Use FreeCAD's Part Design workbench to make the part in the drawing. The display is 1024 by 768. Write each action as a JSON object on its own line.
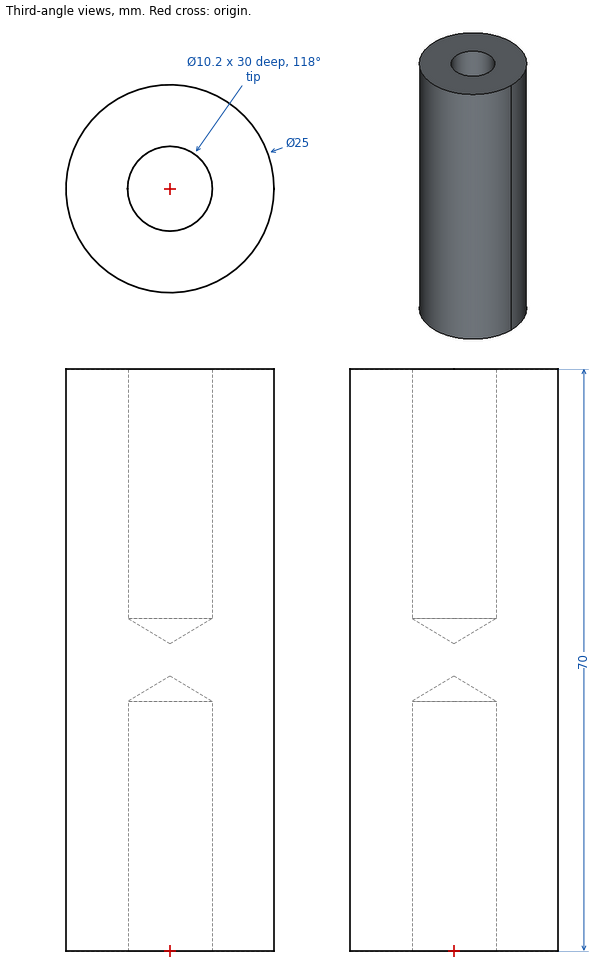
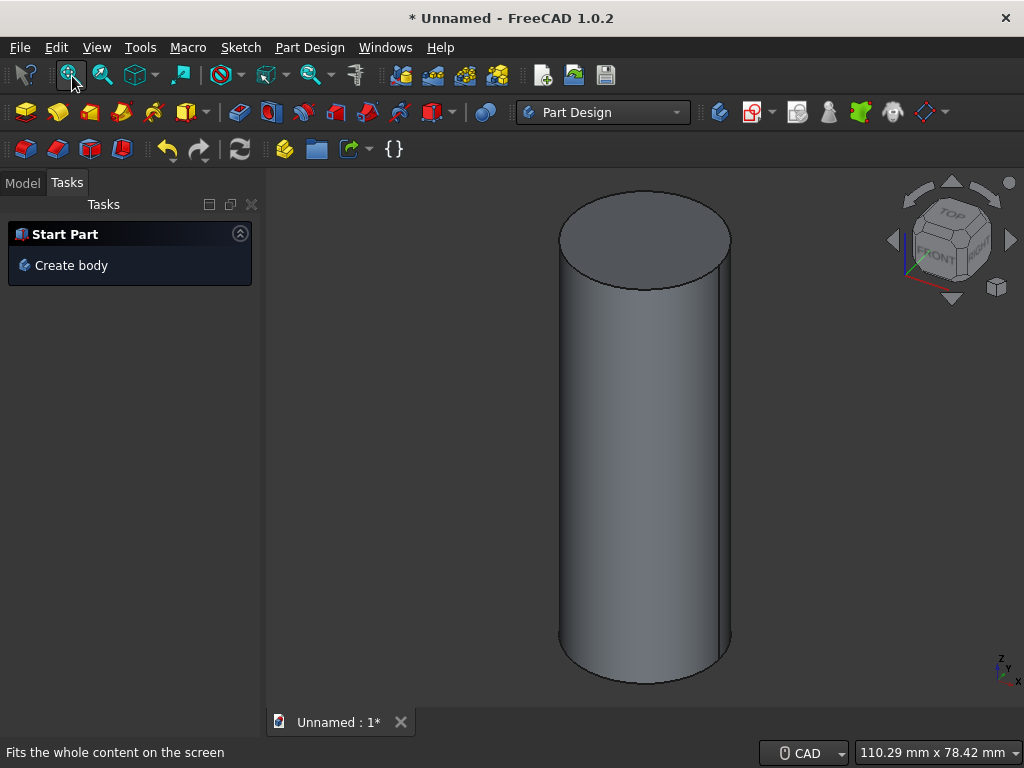
{"action": "left_click", "coordinate": [645, 239]}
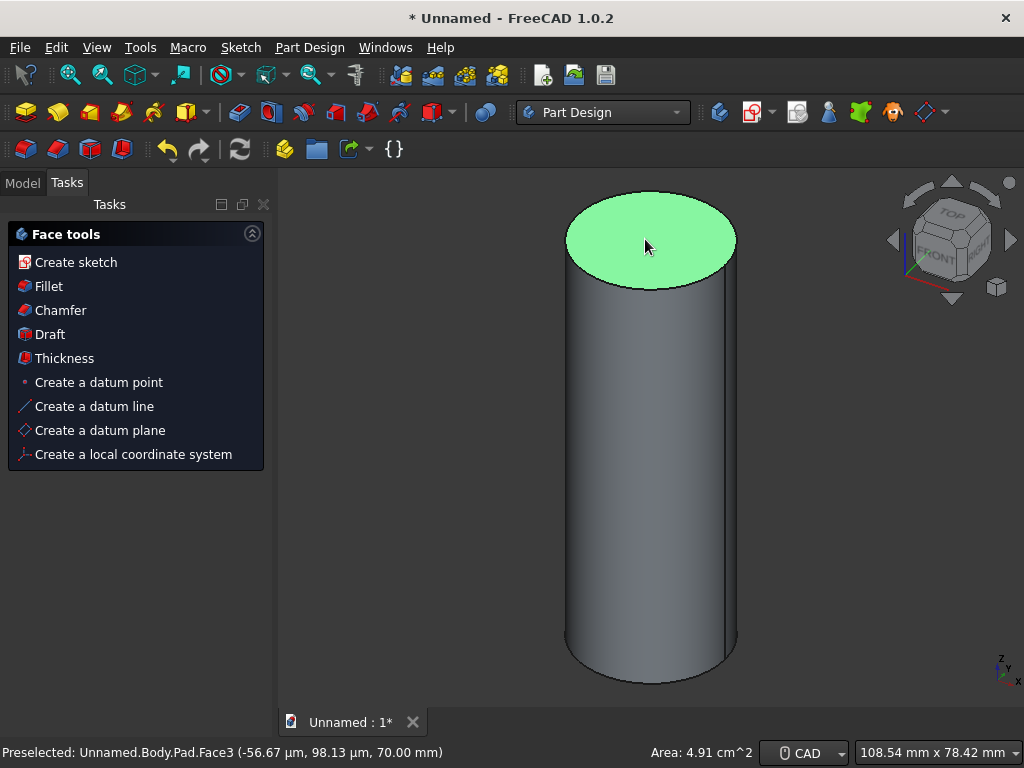
{"action": "left_click", "coordinate": [752, 112]}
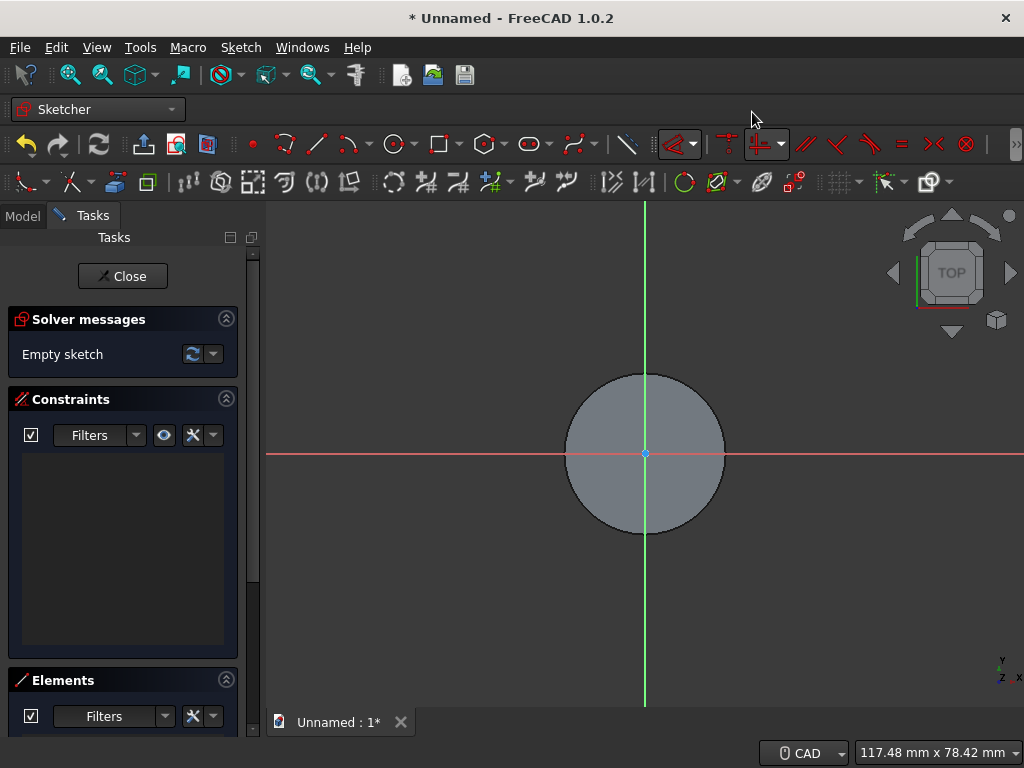
{"action": "scroll", "coordinate": [662, 454], "scroll_direction": "up", "scroll_amount": 8}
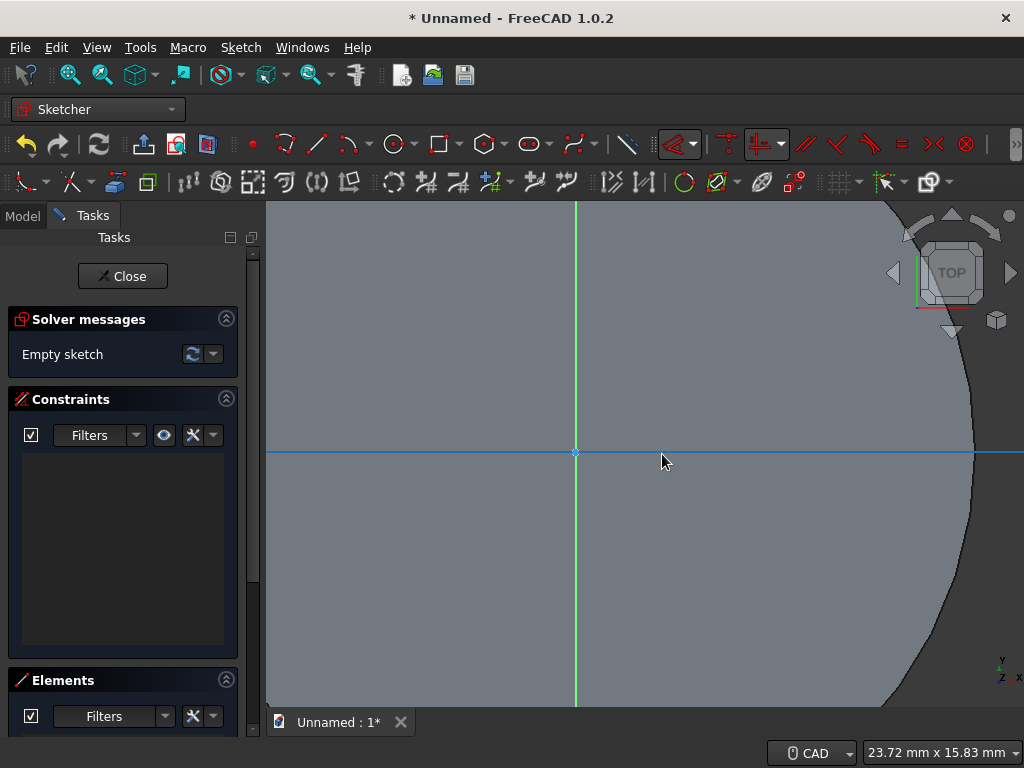
{"action": "key", "text": "g c"}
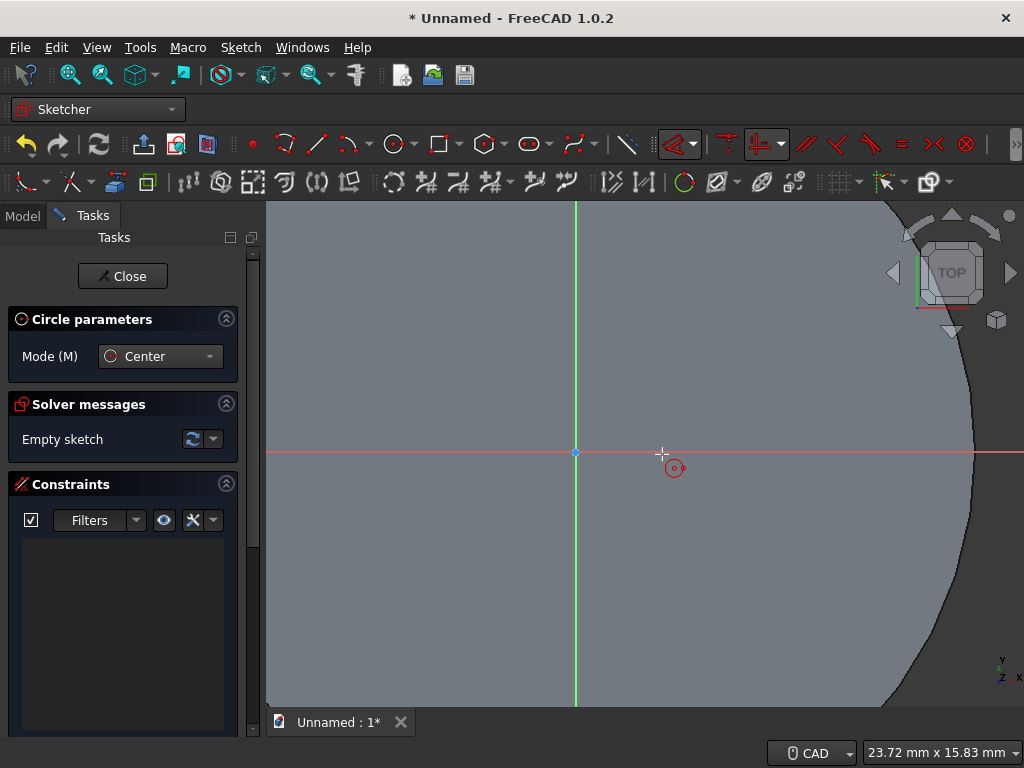
{"action": "left_click", "coordinate": [576, 452]}
{"action": "mouse_move", "coordinate": [691, 337]}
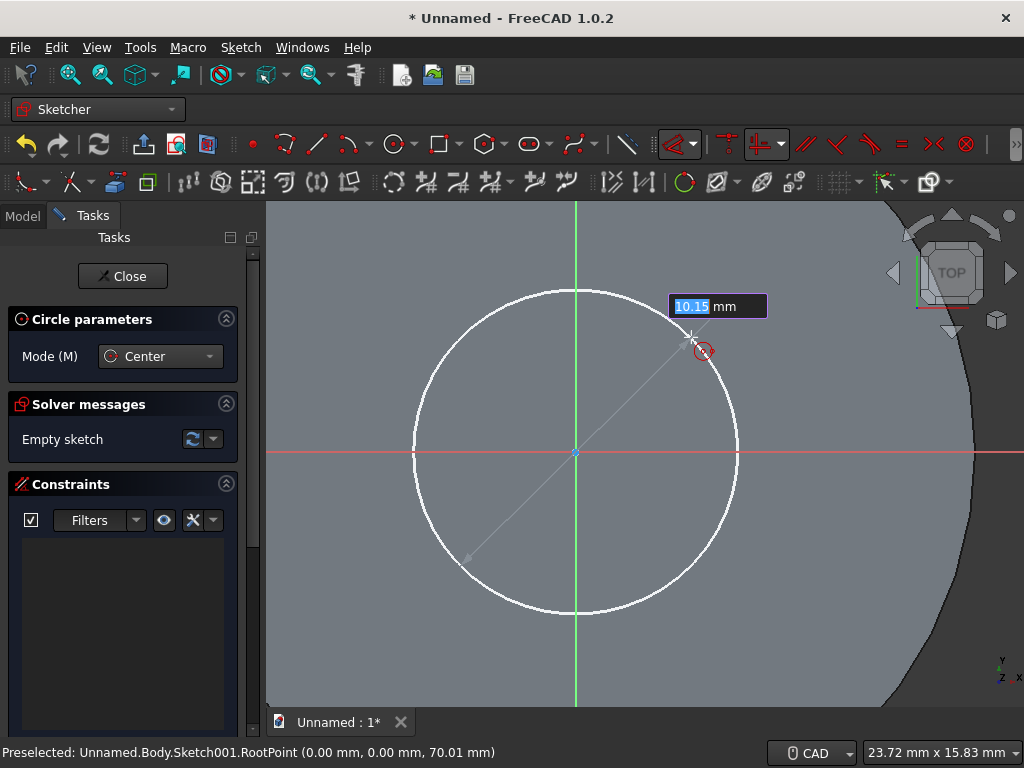
{"action": "type", "text": "10.2"}
{"action": "key", "text": "Return"}
{"action": "key", "text": "Escape"}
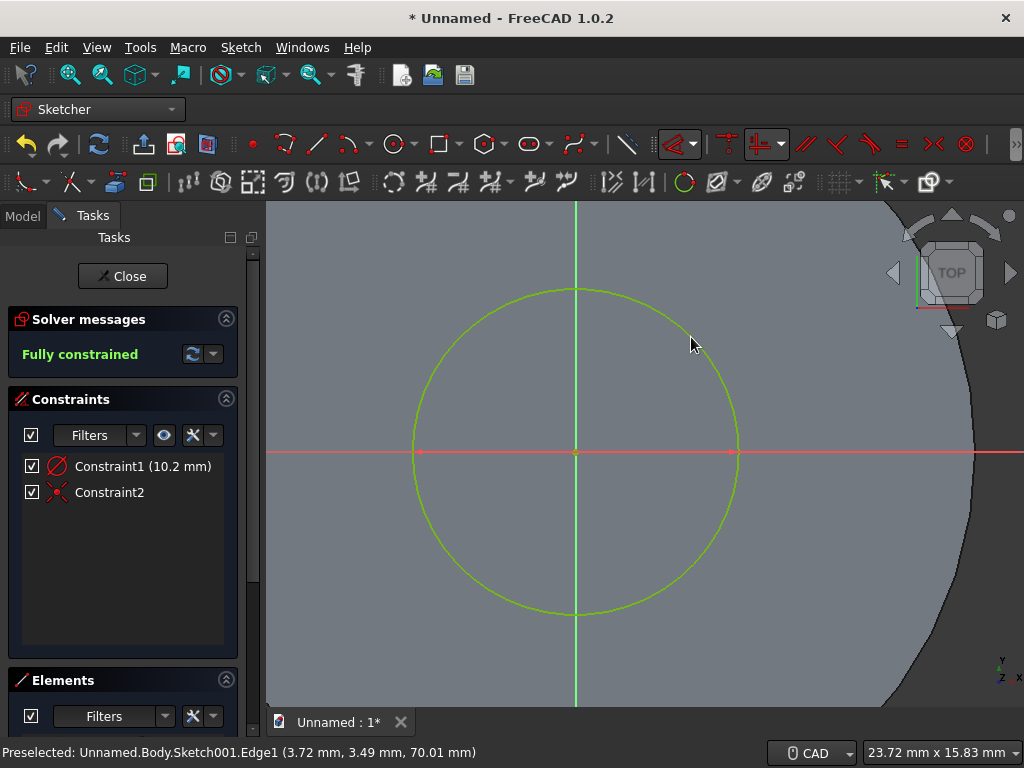
{"action": "left_click", "coordinate": [123, 276]}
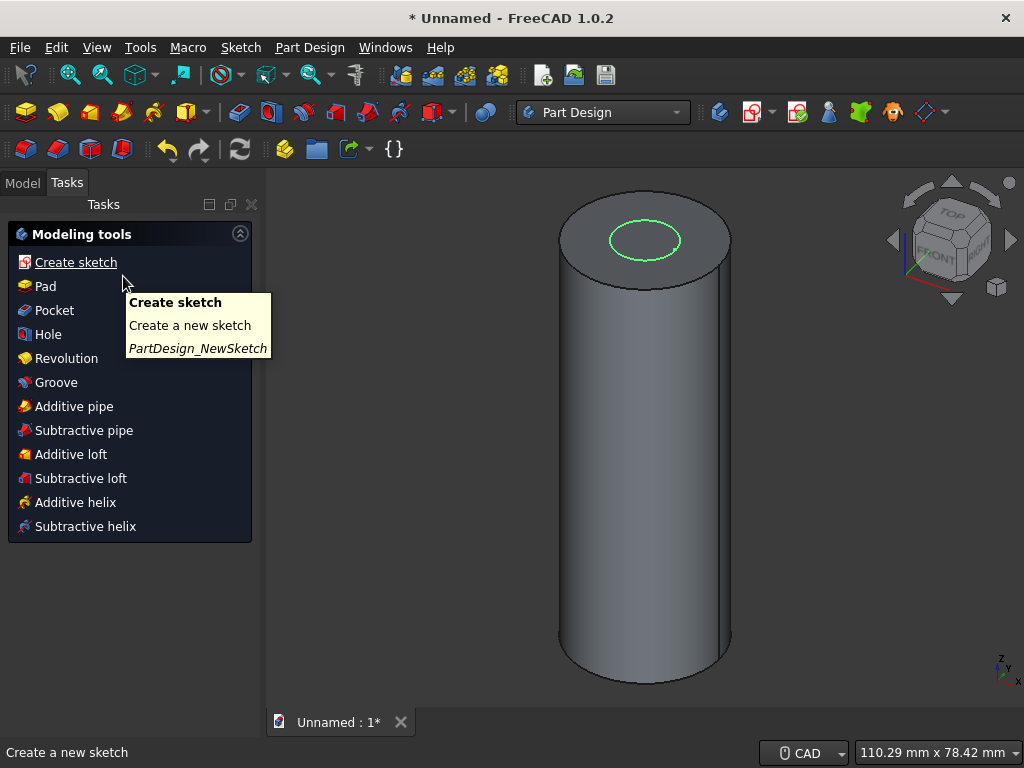
{"action": "left_click", "coordinate": [272, 112]}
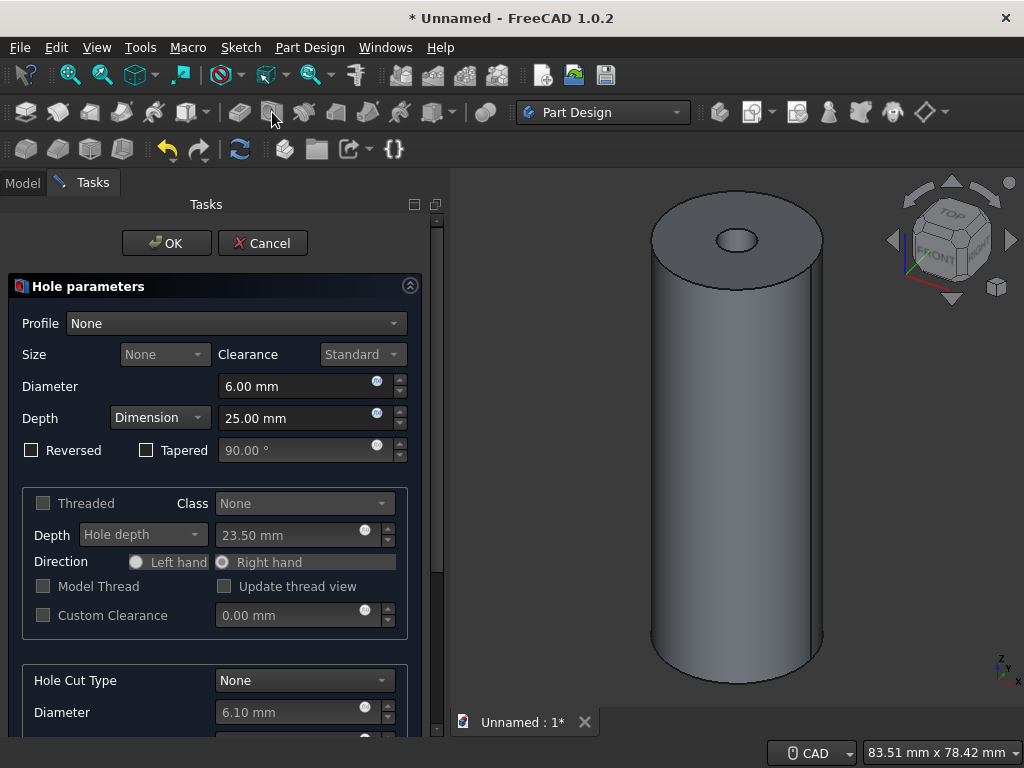
{"action": "triple_click", "coordinate": [305, 386]}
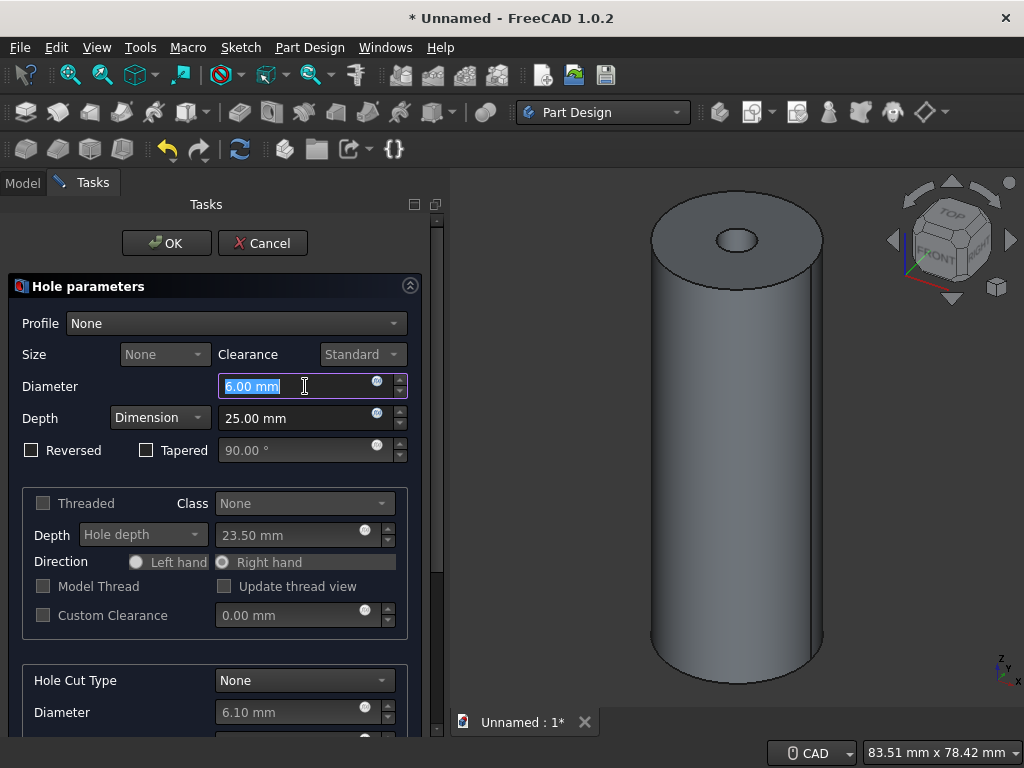
{"action": "type", "text": "10.2"}
{"action": "key", "text": "Tab"}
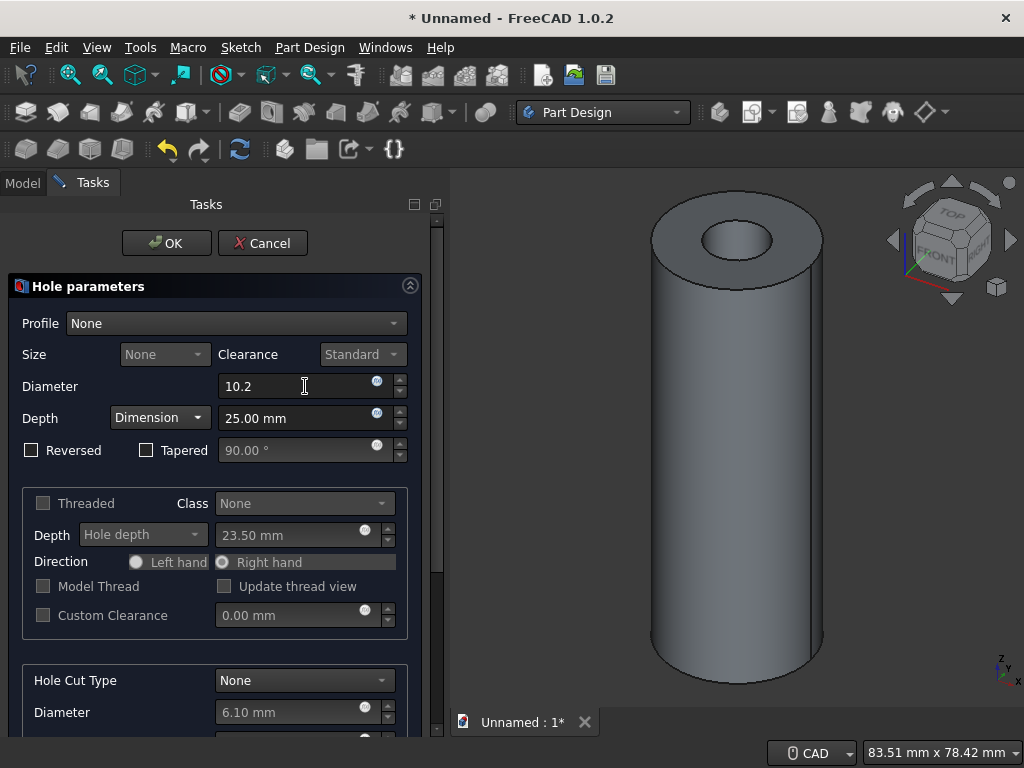
{"action": "triple_click", "coordinate": [305, 418]}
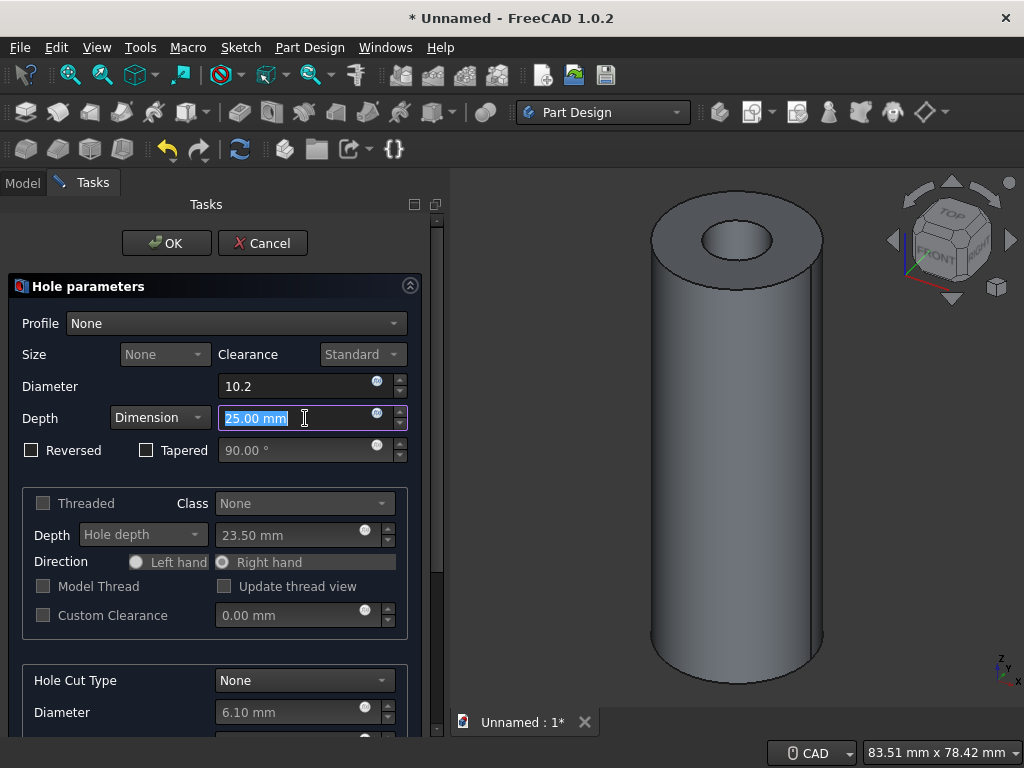
{"action": "type", "text": "30"}
{"action": "key", "text": "Tab"}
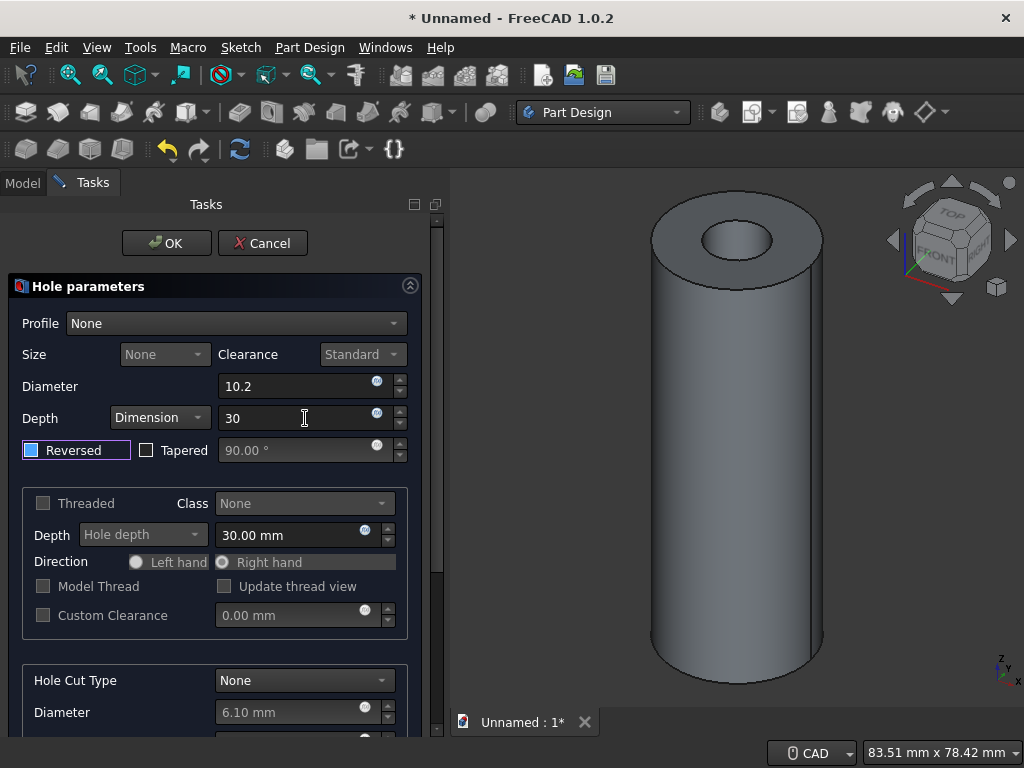
{"action": "left_click", "coordinate": [167, 243]}